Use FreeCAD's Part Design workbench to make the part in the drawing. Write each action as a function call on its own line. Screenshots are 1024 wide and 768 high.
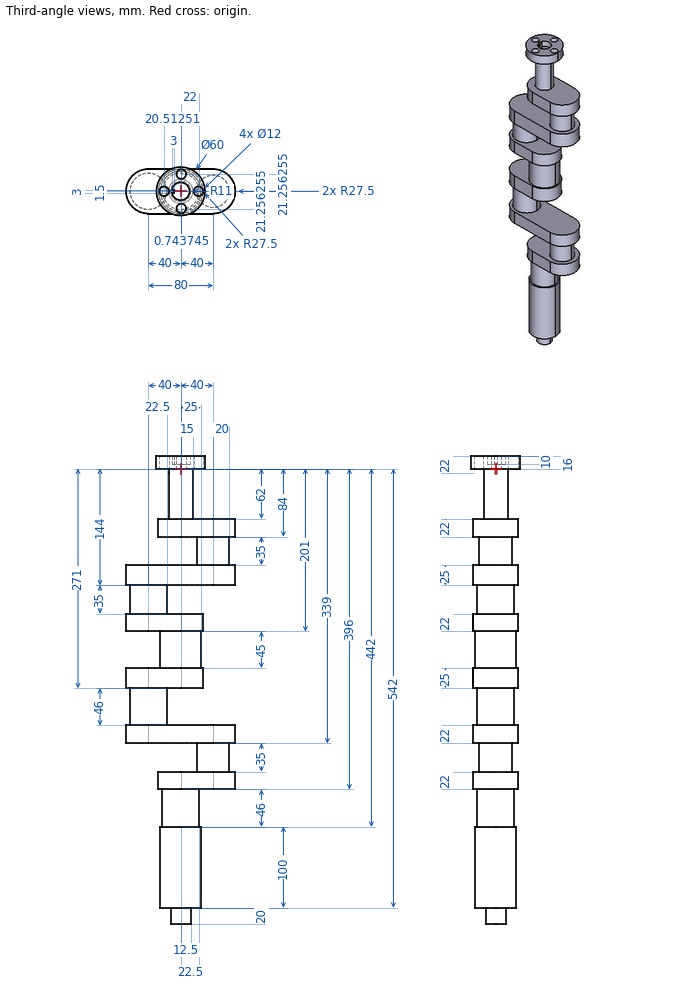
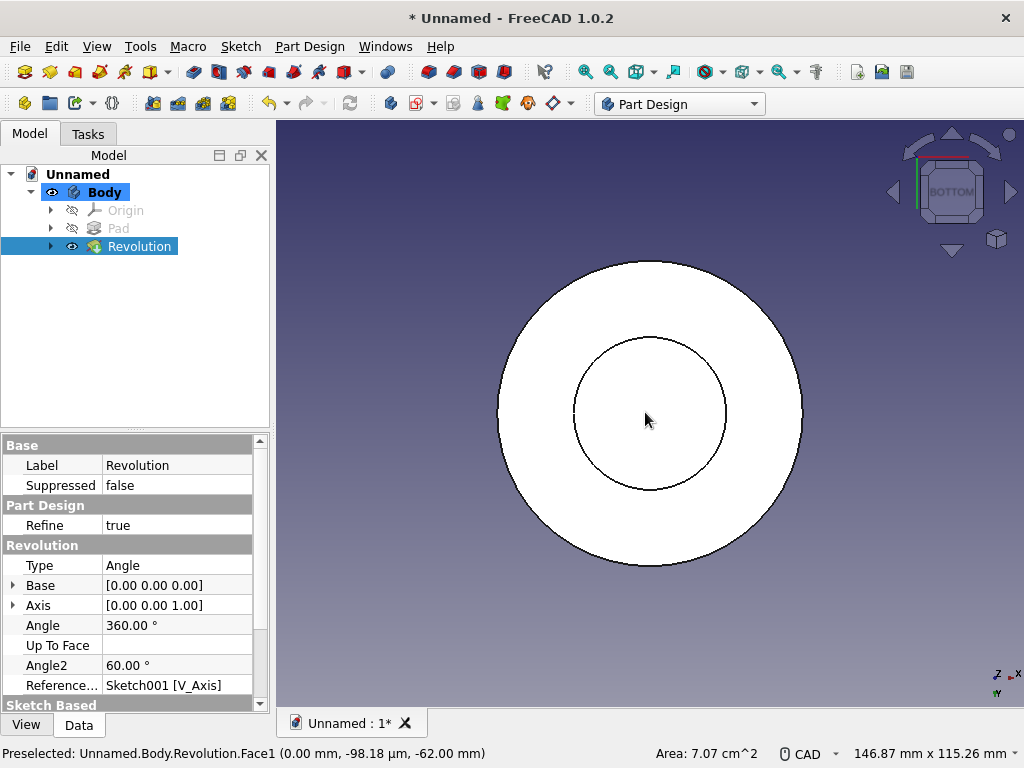
click(416, 104)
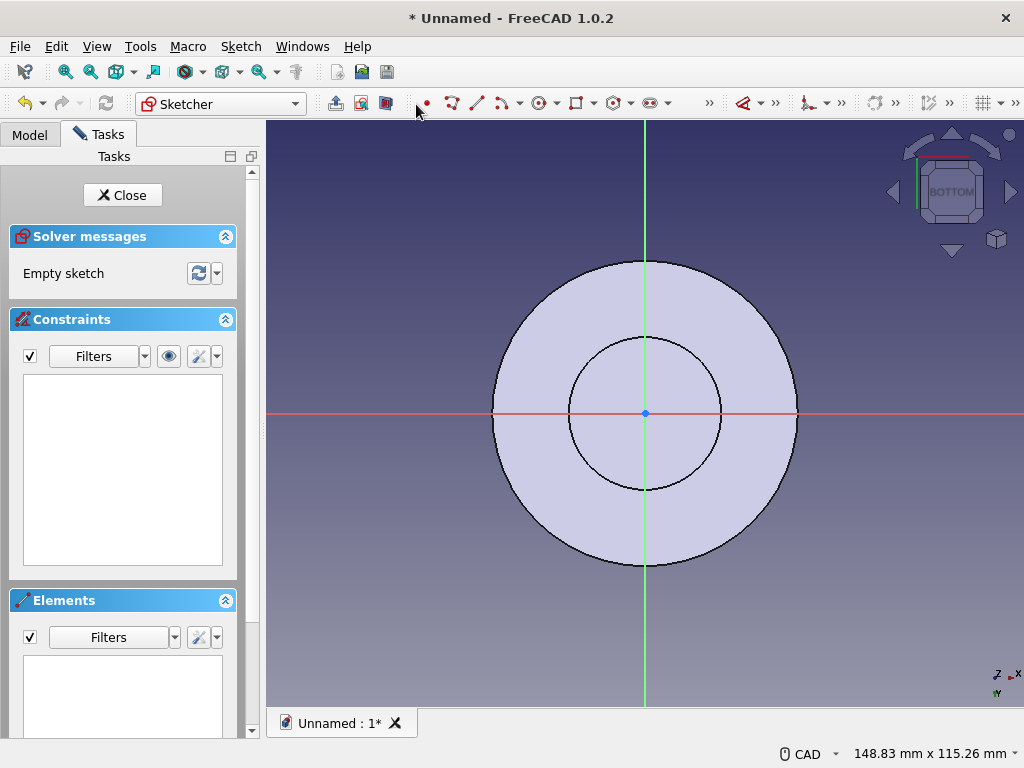
scroll(294, 414, down, 2)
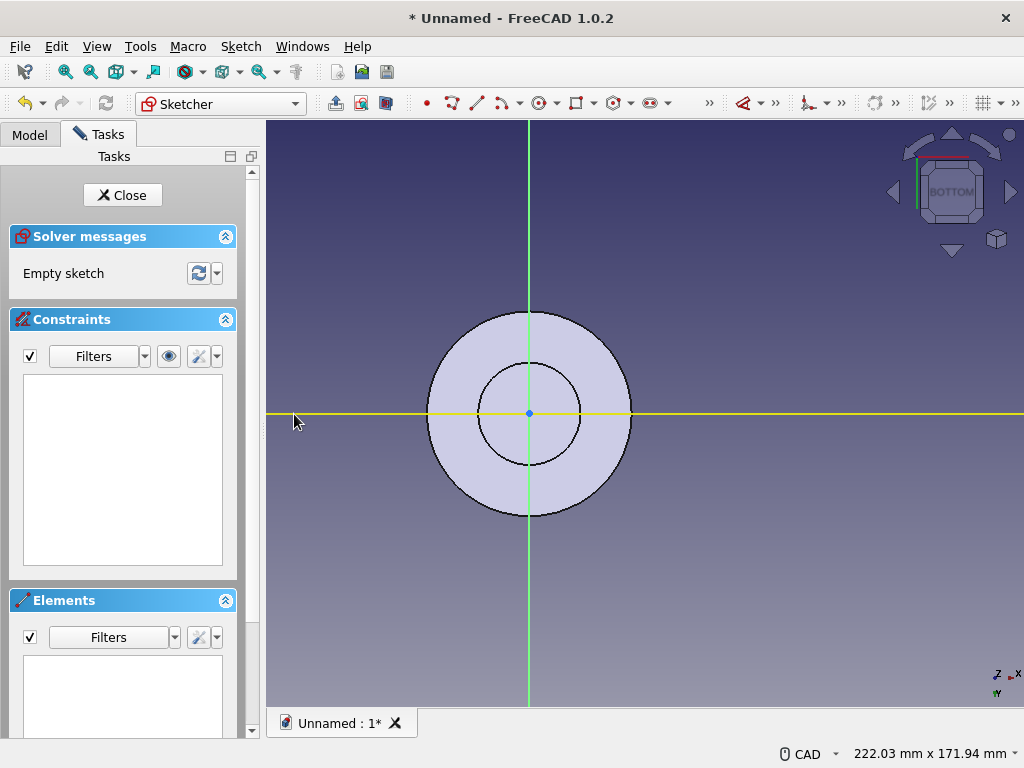
key(g)
key(s)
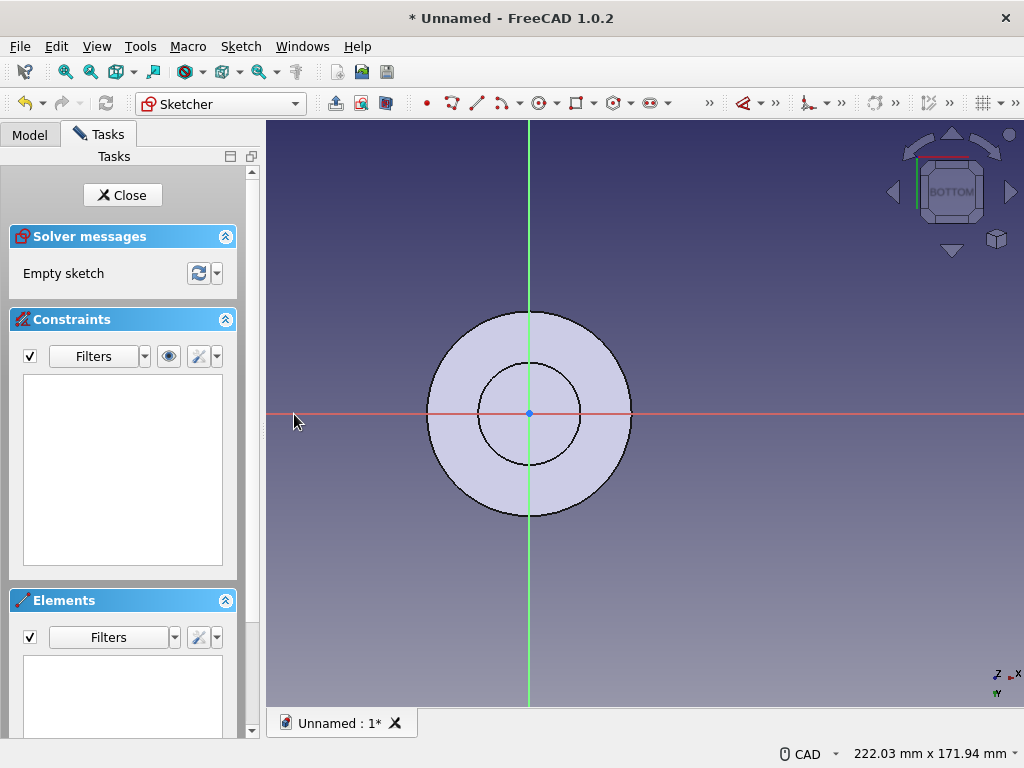
click(529, 414)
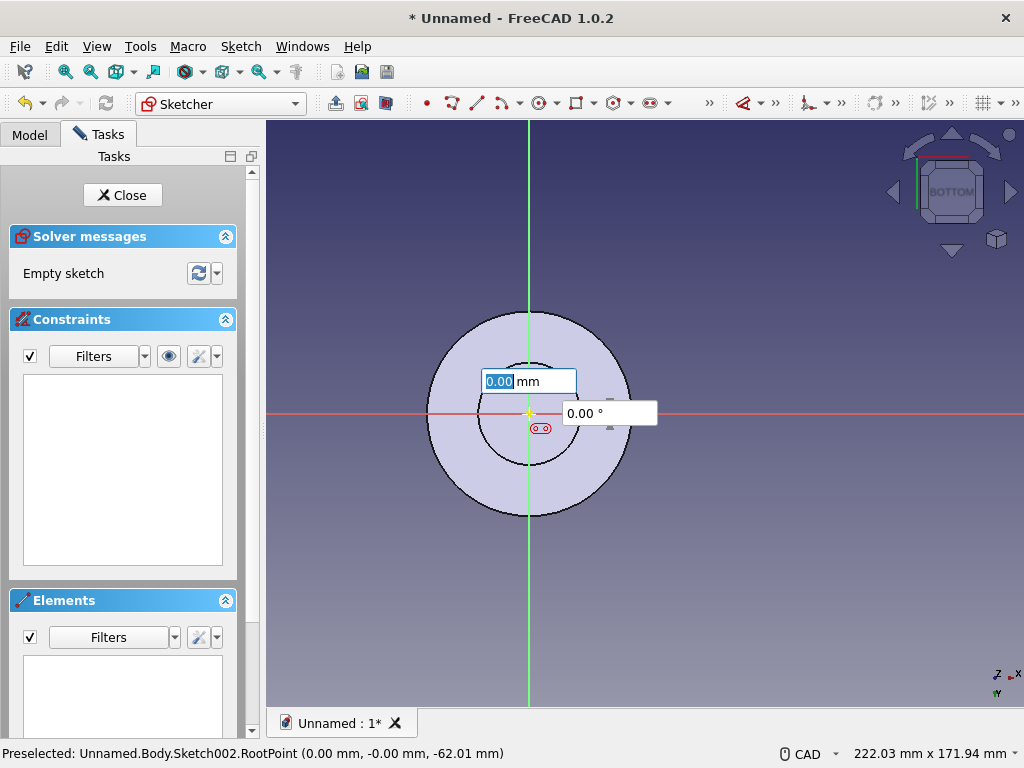
click(666, 405)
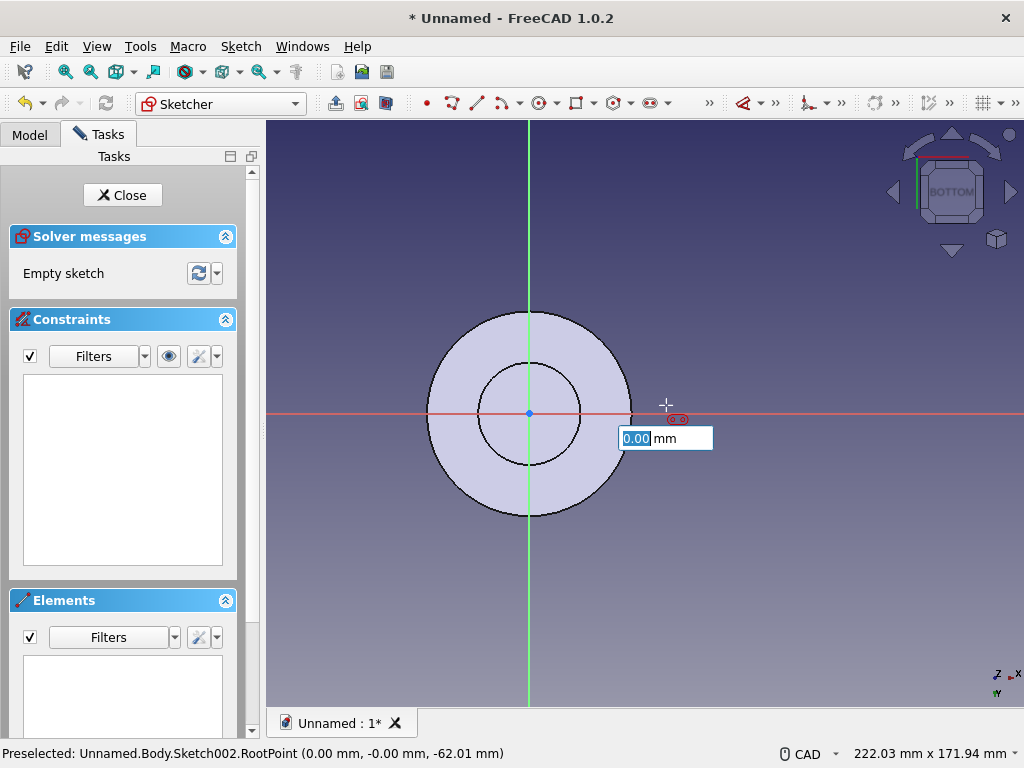
click(598, 508)
key(Escape)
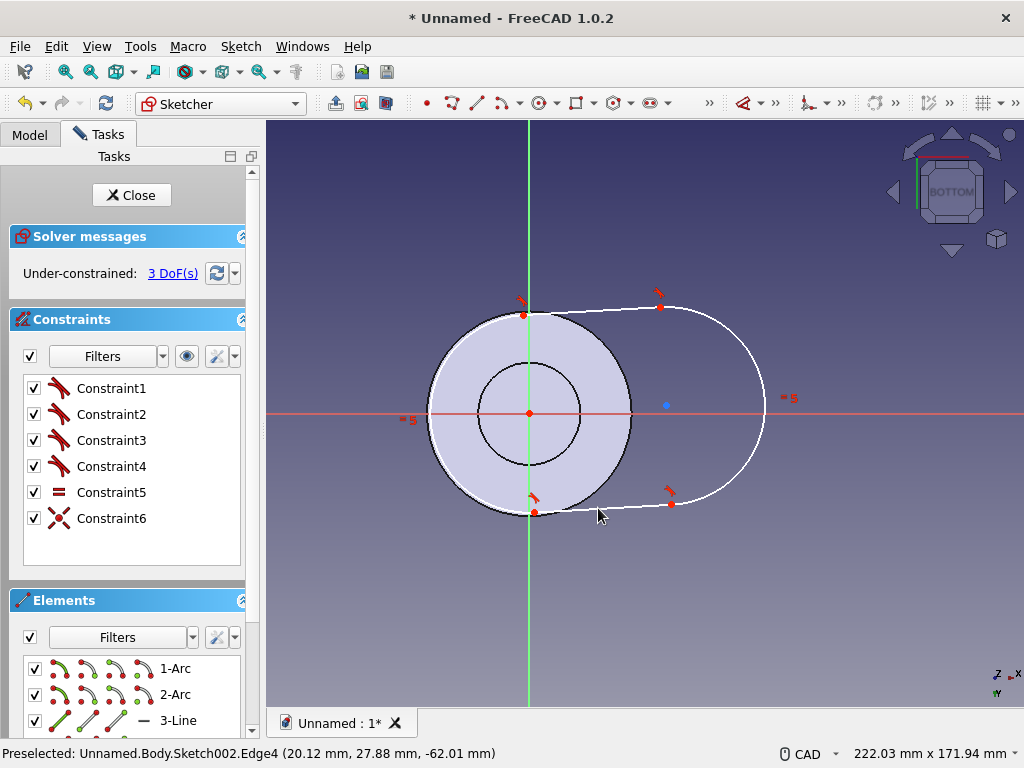
click(565, 313)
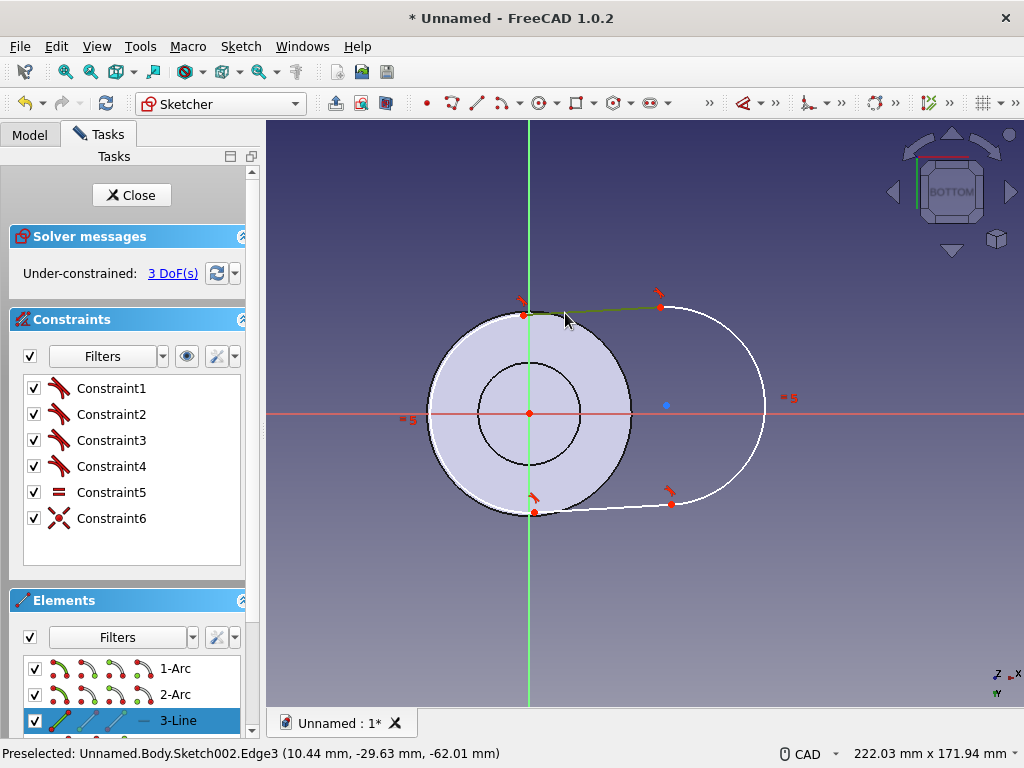
key(h)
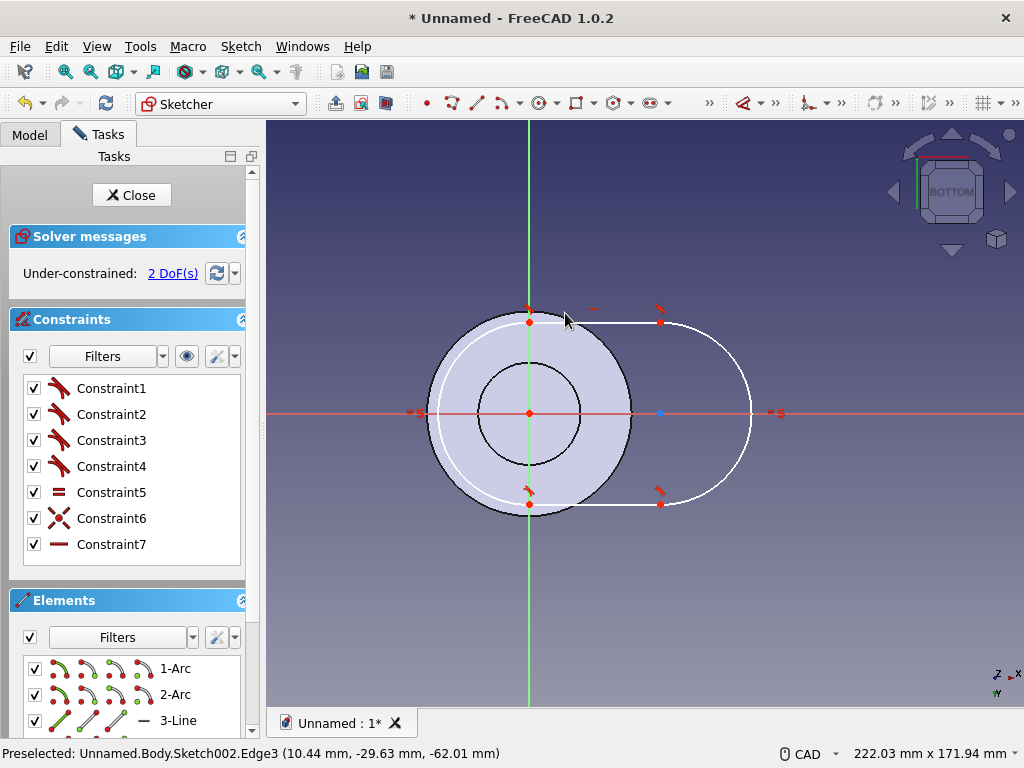
click(742, 104)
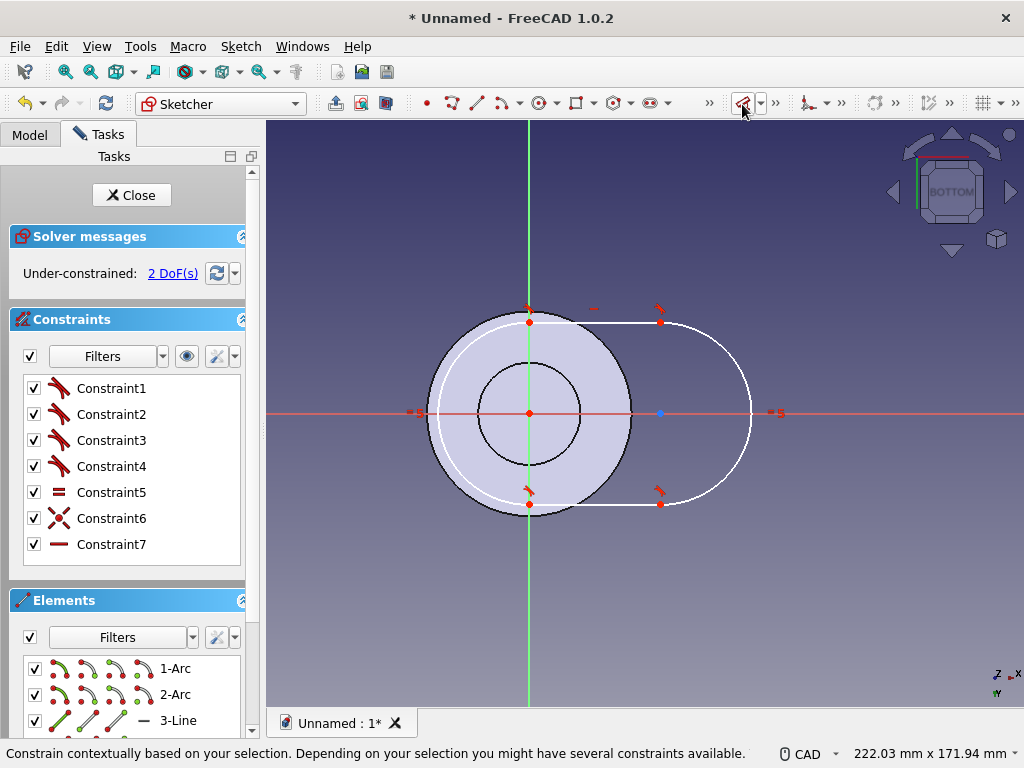
click(456, 360)
click(430, 341)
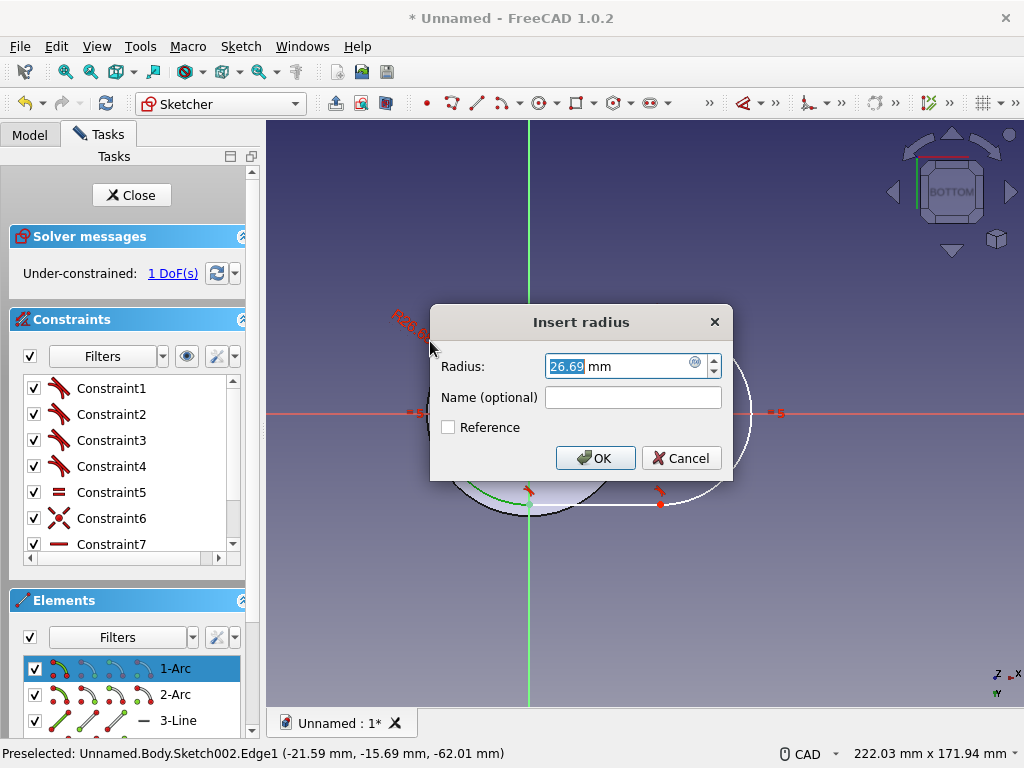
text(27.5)
key(Return)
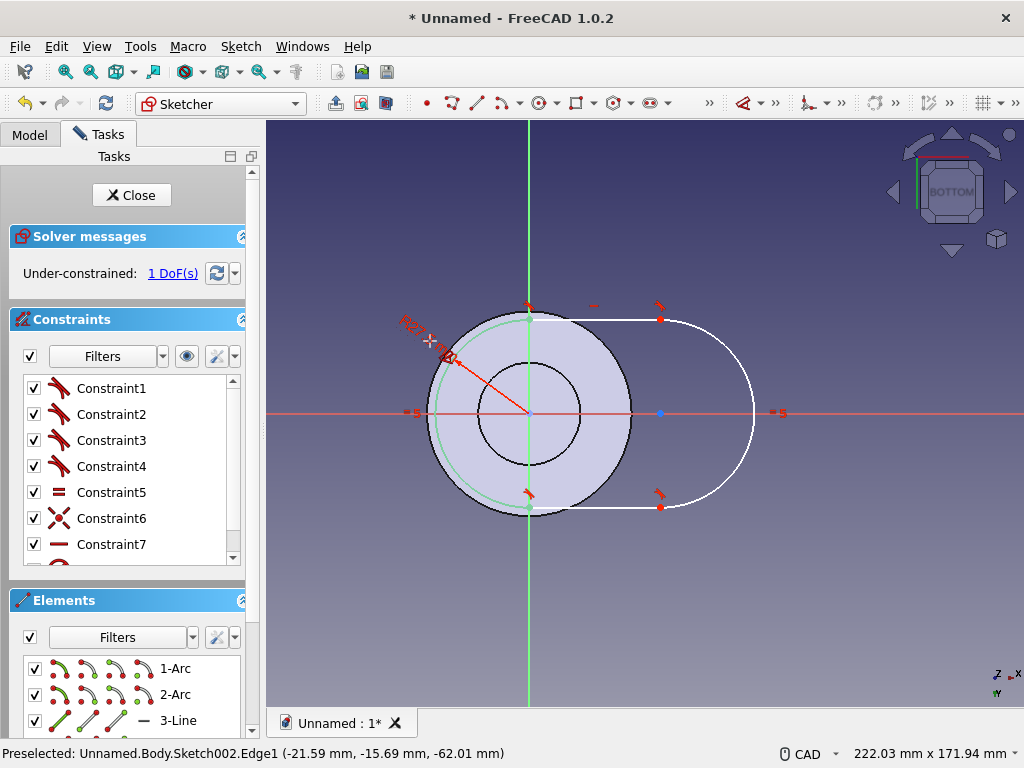
click(569, 320)
click(595, 286)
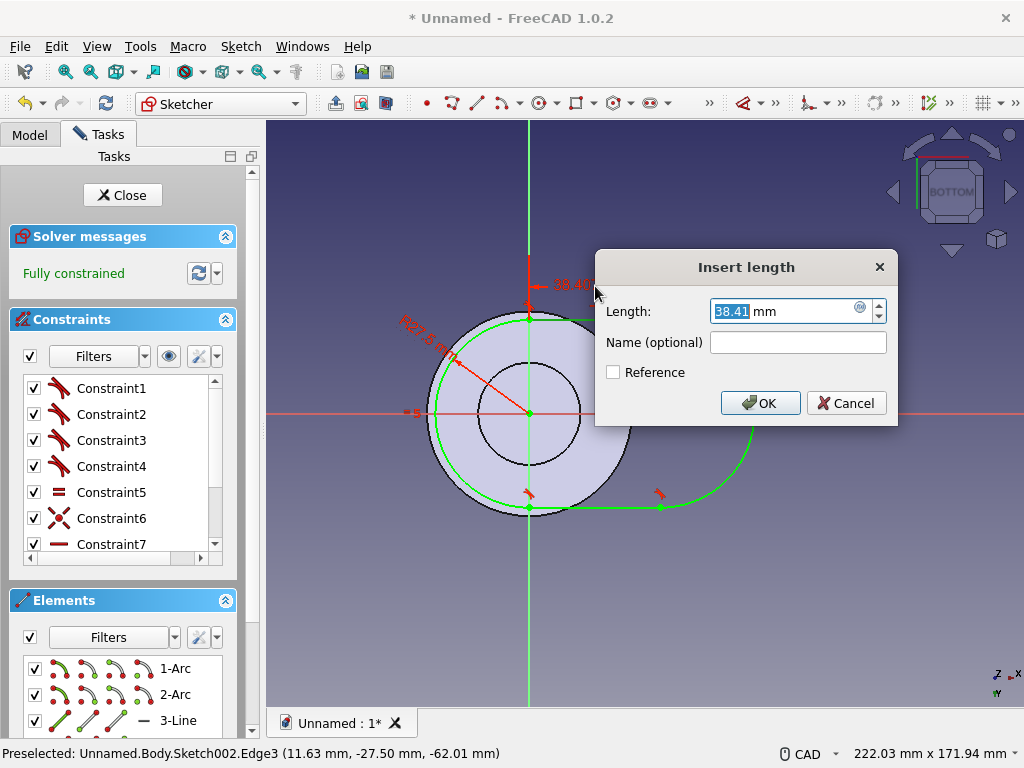
text(40)
key(Return)
key(Escape)